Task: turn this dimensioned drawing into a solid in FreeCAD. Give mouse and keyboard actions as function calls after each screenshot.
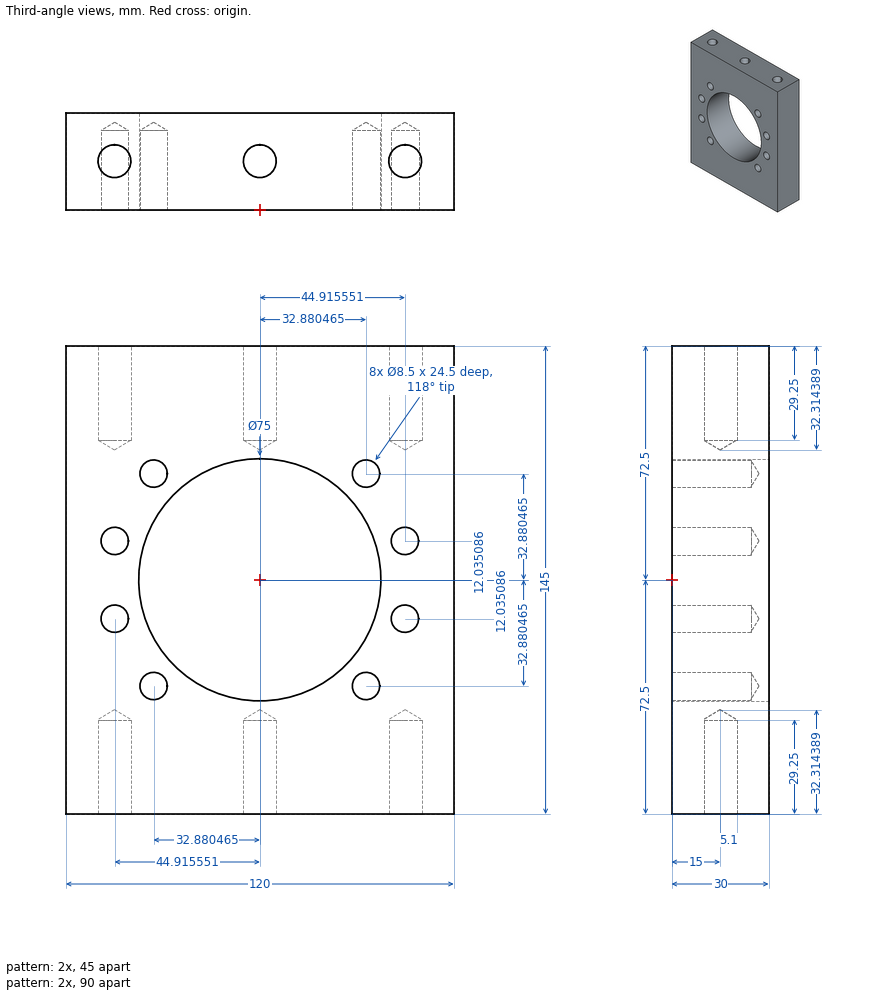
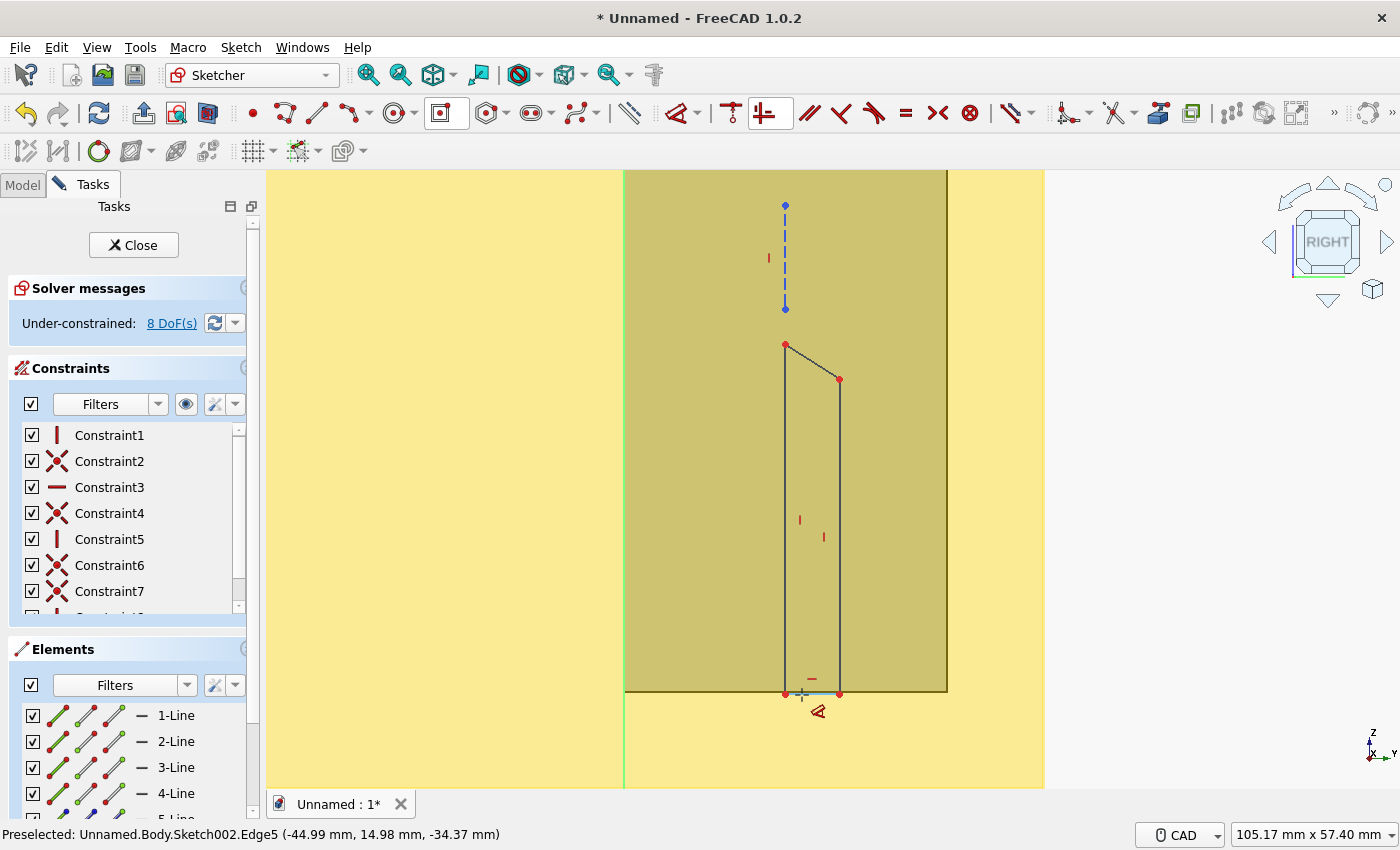
click(802, 694)
click(813, 728)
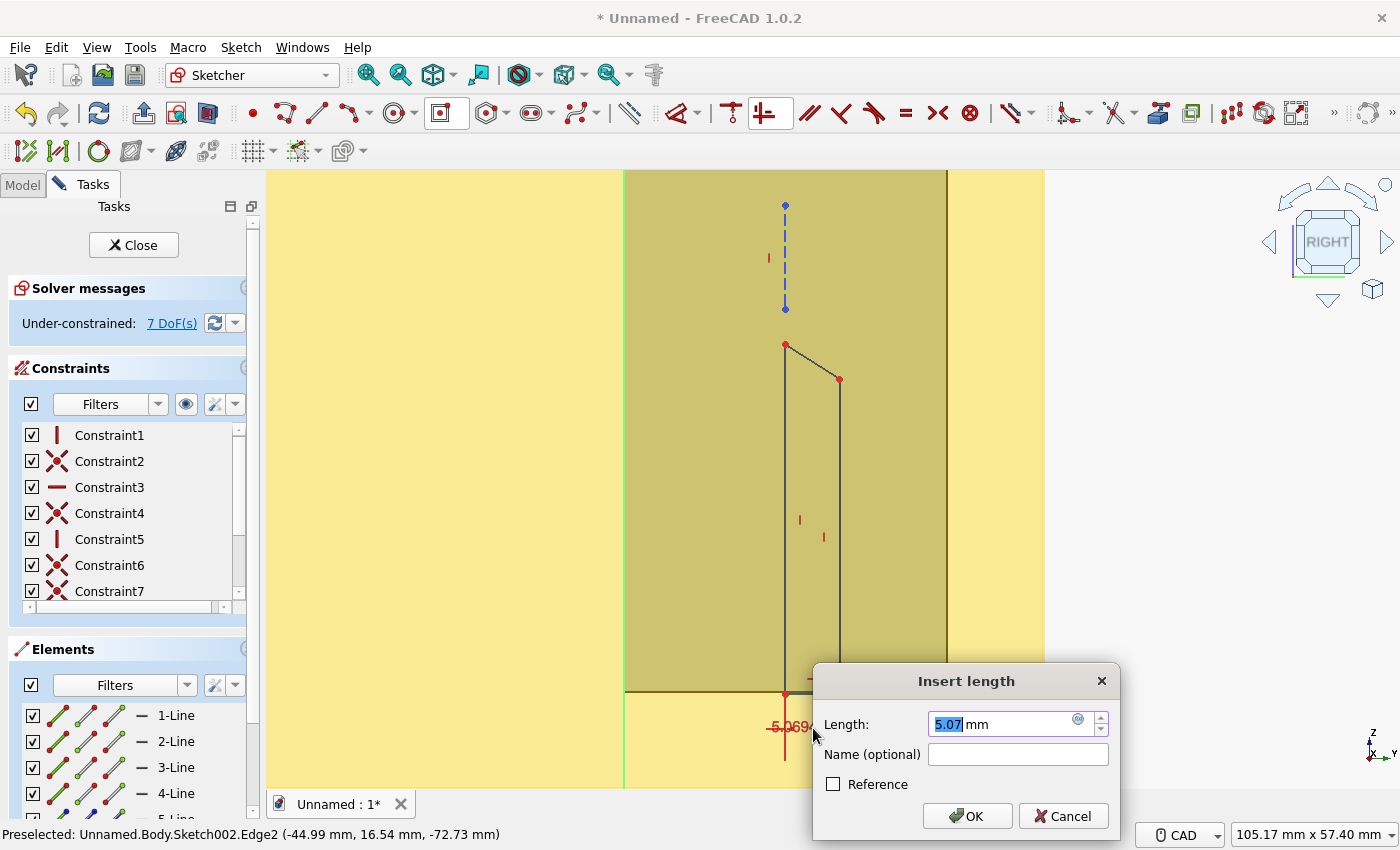
text(5.1)
key(Return)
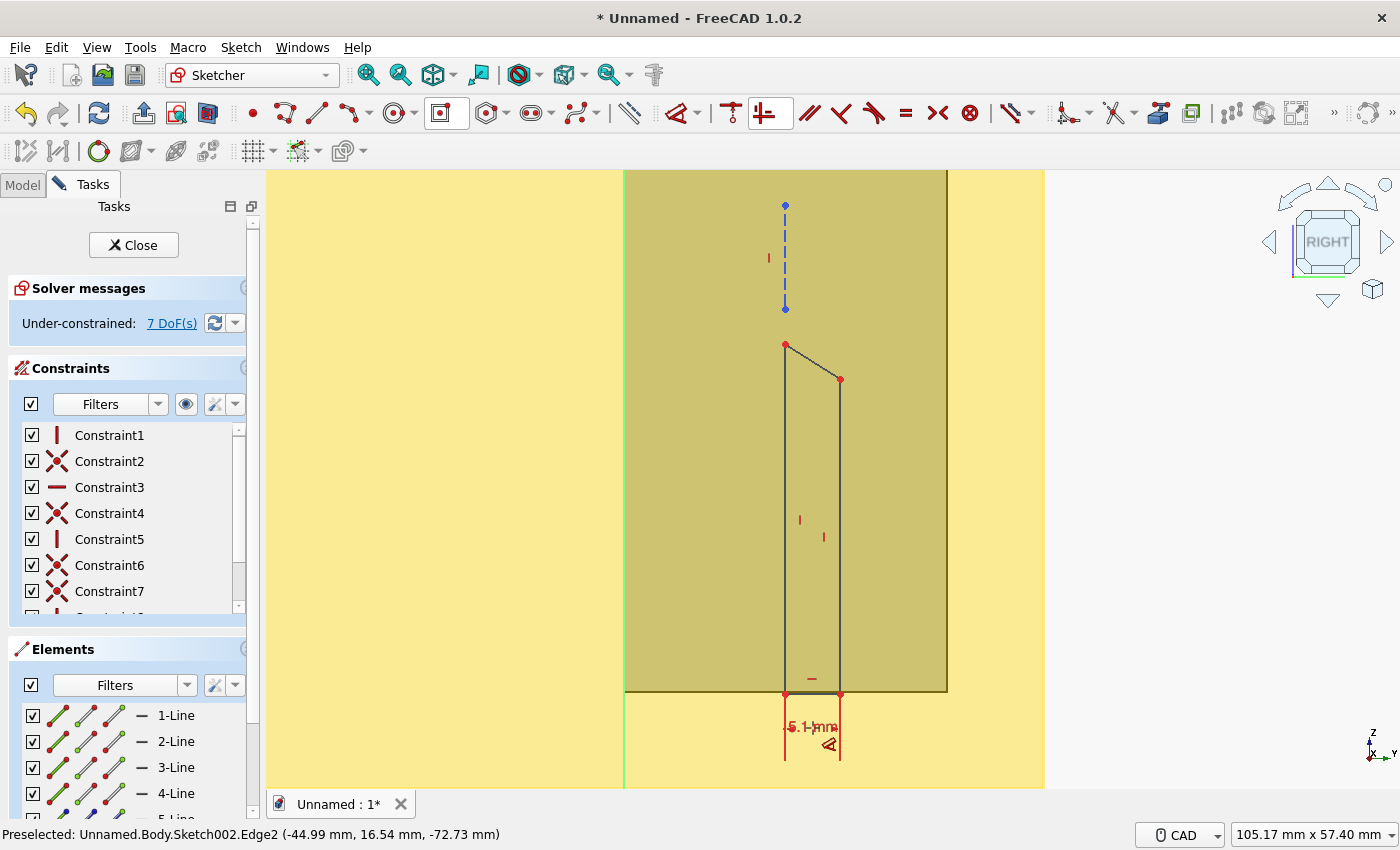
click(785, 344)
click(704, 378)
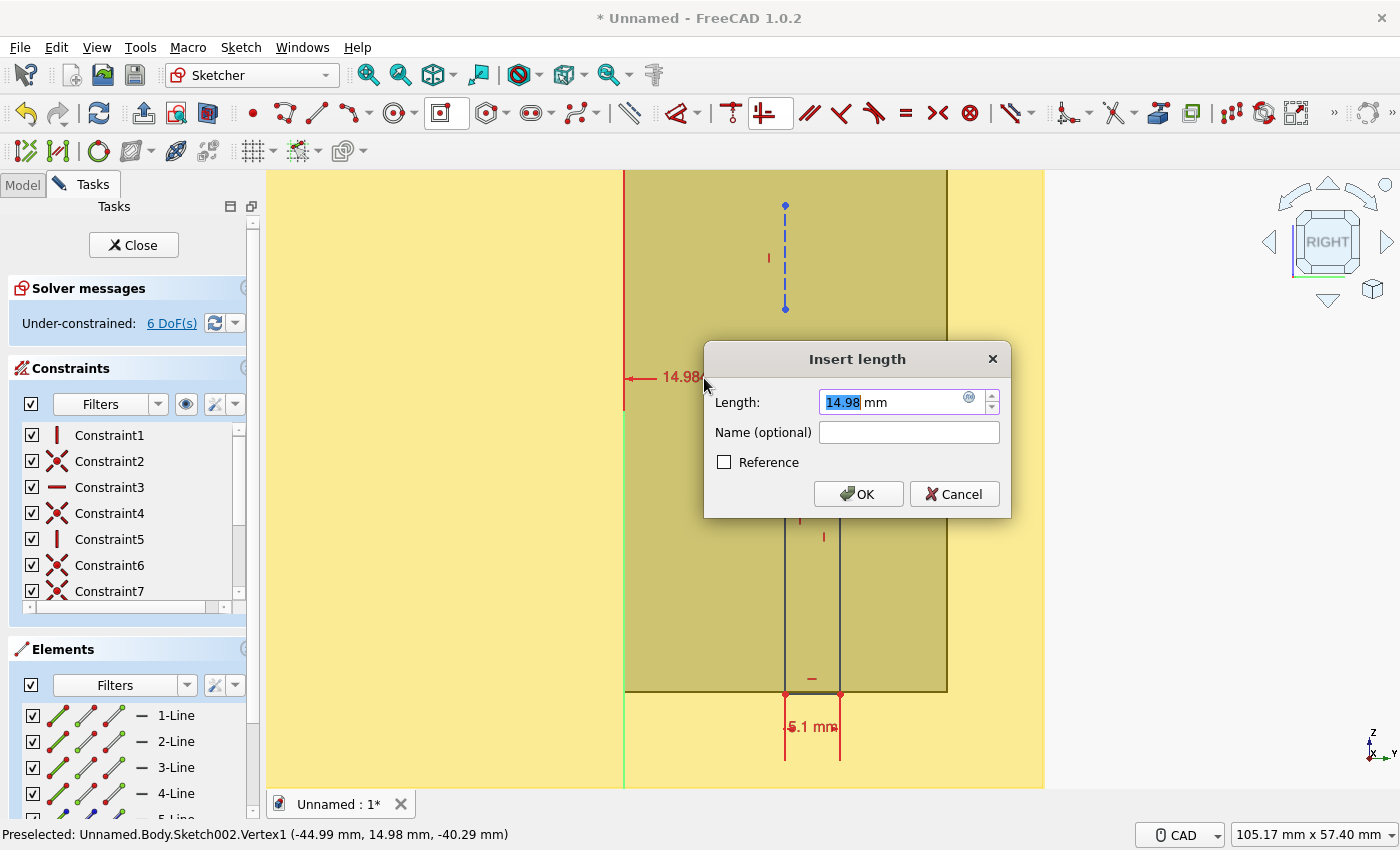
text(15)
key(Return)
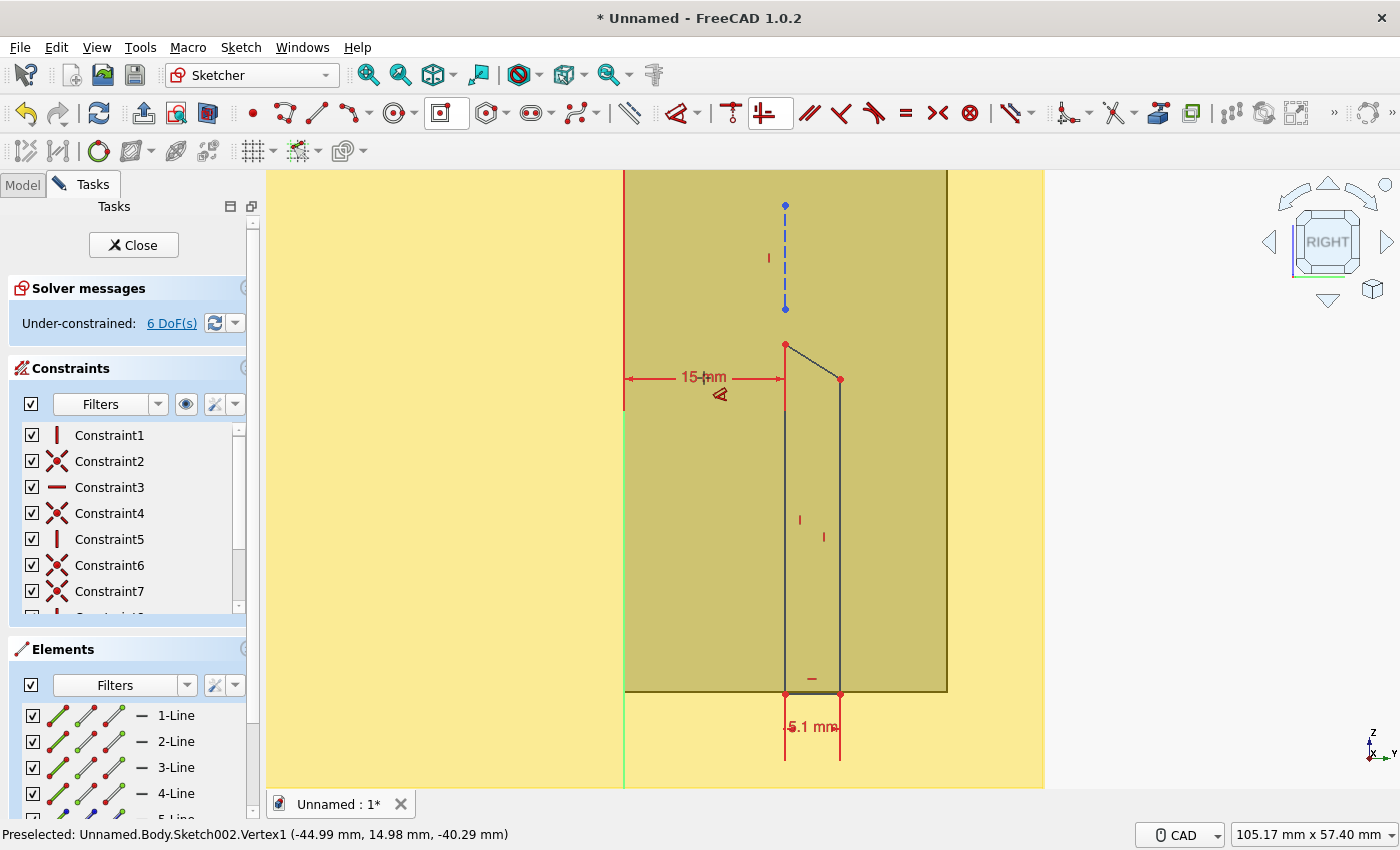
click(785, 310)
click(704, 344)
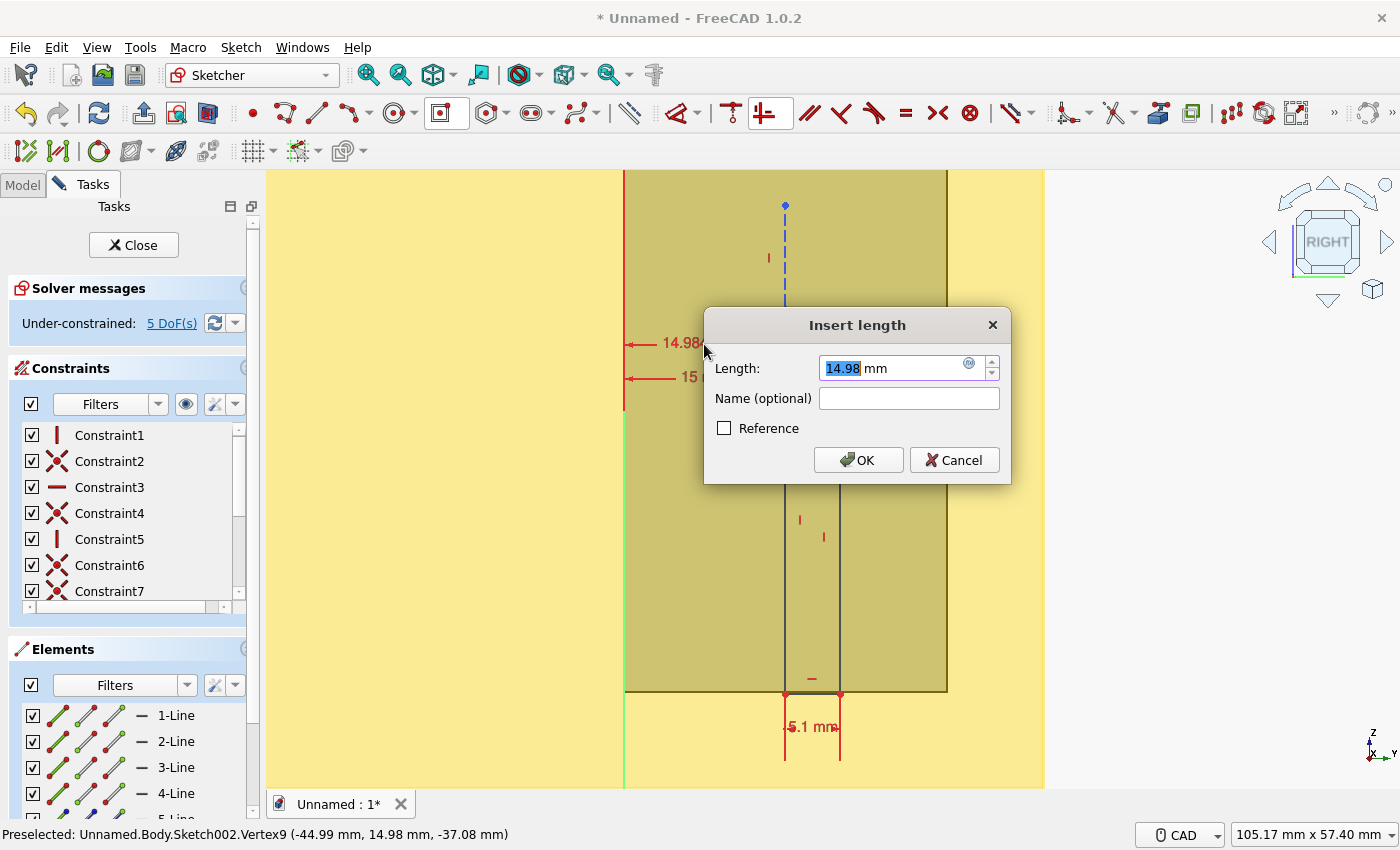
text(15)
key(Return)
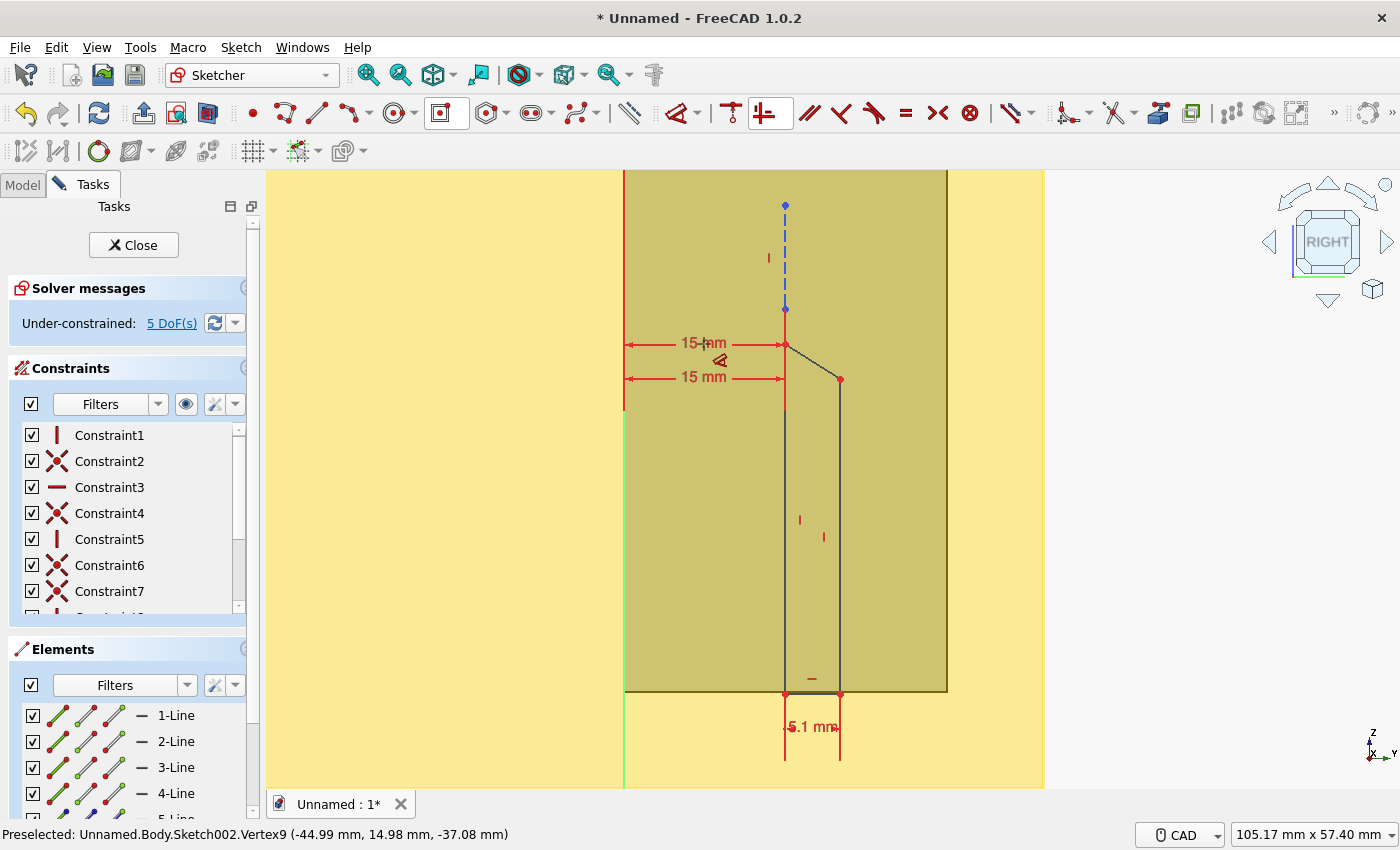
click(840, 600)
click(874, 537)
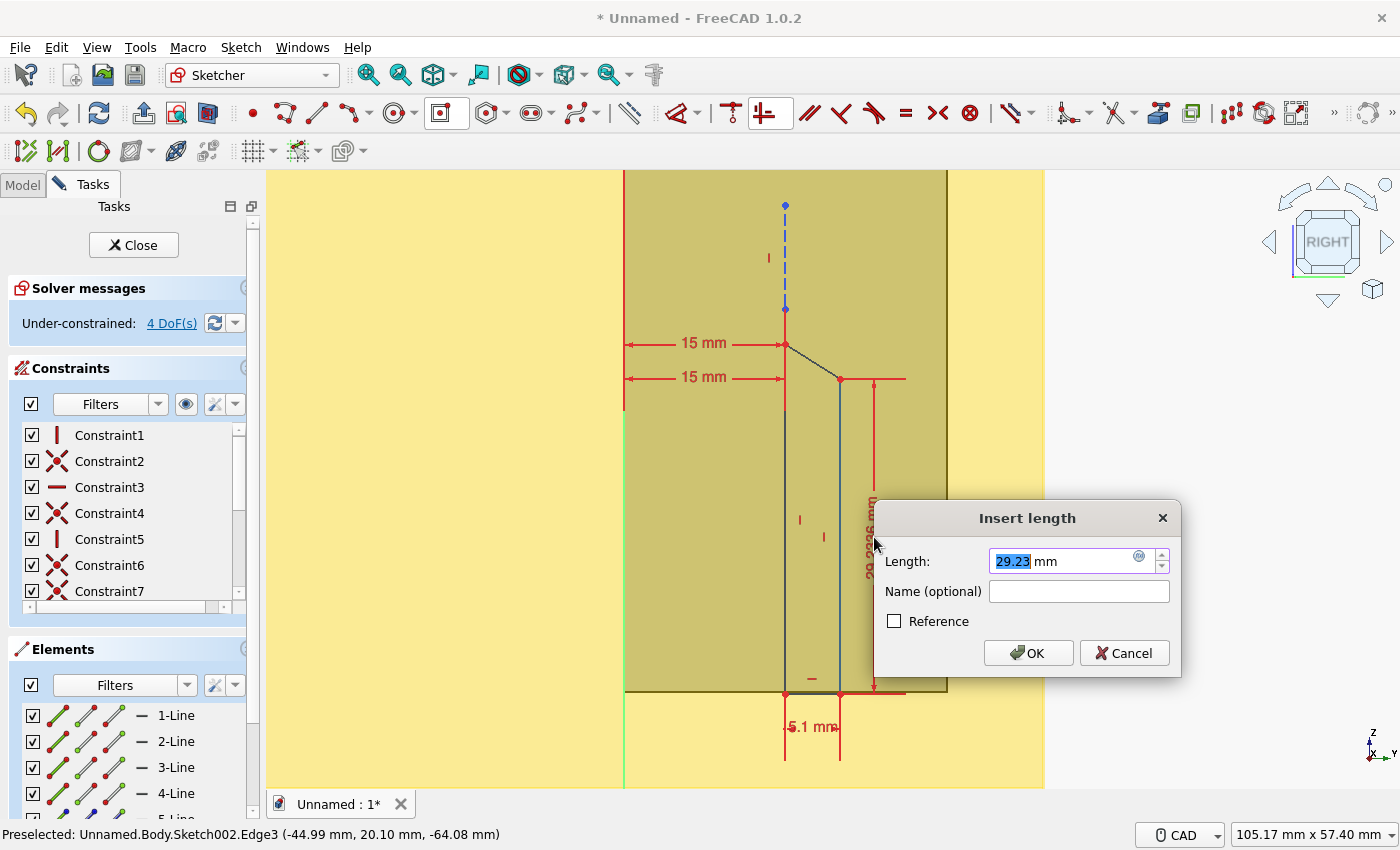
text(29.25)
key(Return)